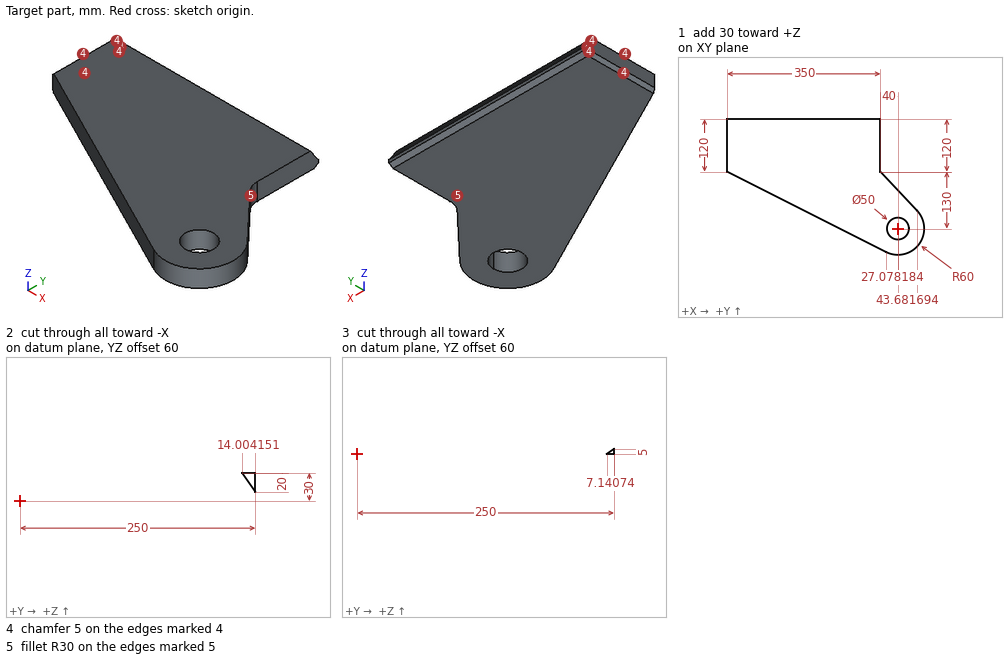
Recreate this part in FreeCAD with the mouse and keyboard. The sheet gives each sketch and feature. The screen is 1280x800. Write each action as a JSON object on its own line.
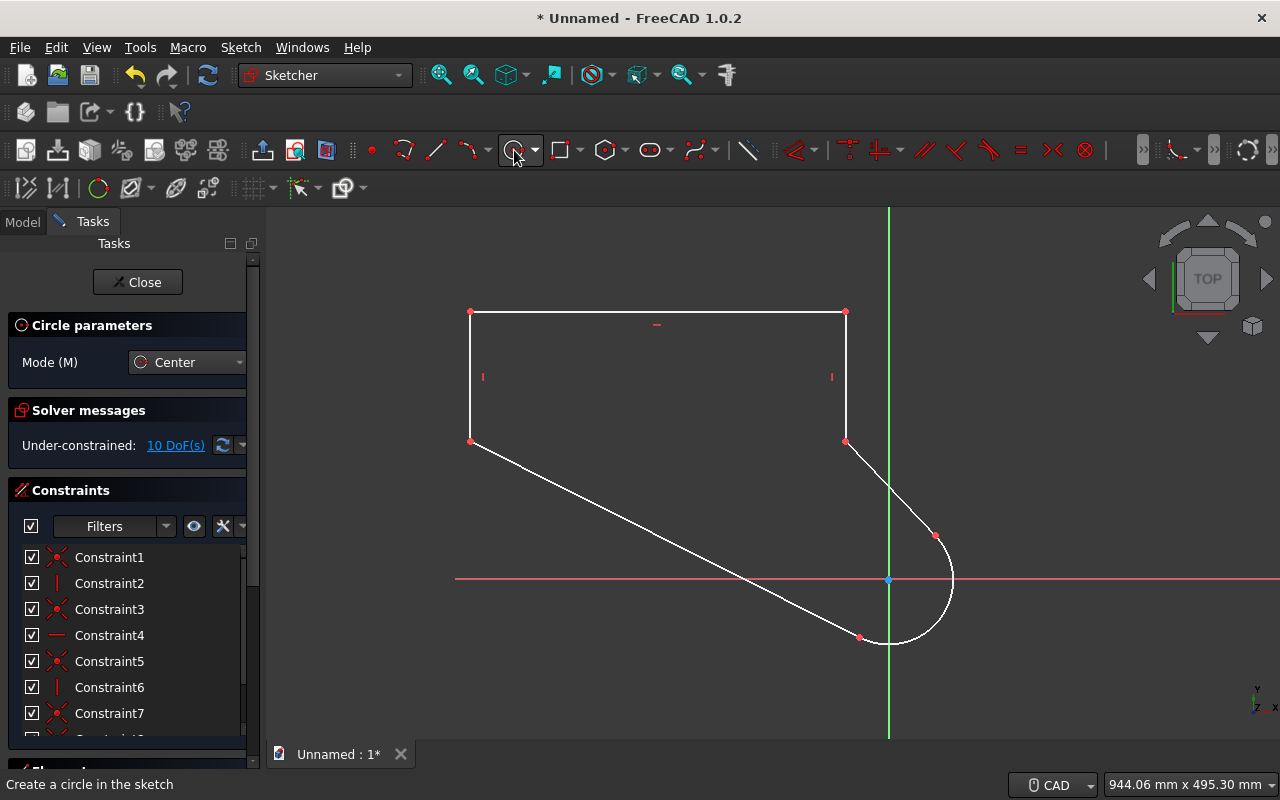
{"action": "left_click", "coordinate": [889, 579]}
{"action": "mouse_move", "coordinate": [908, 560]}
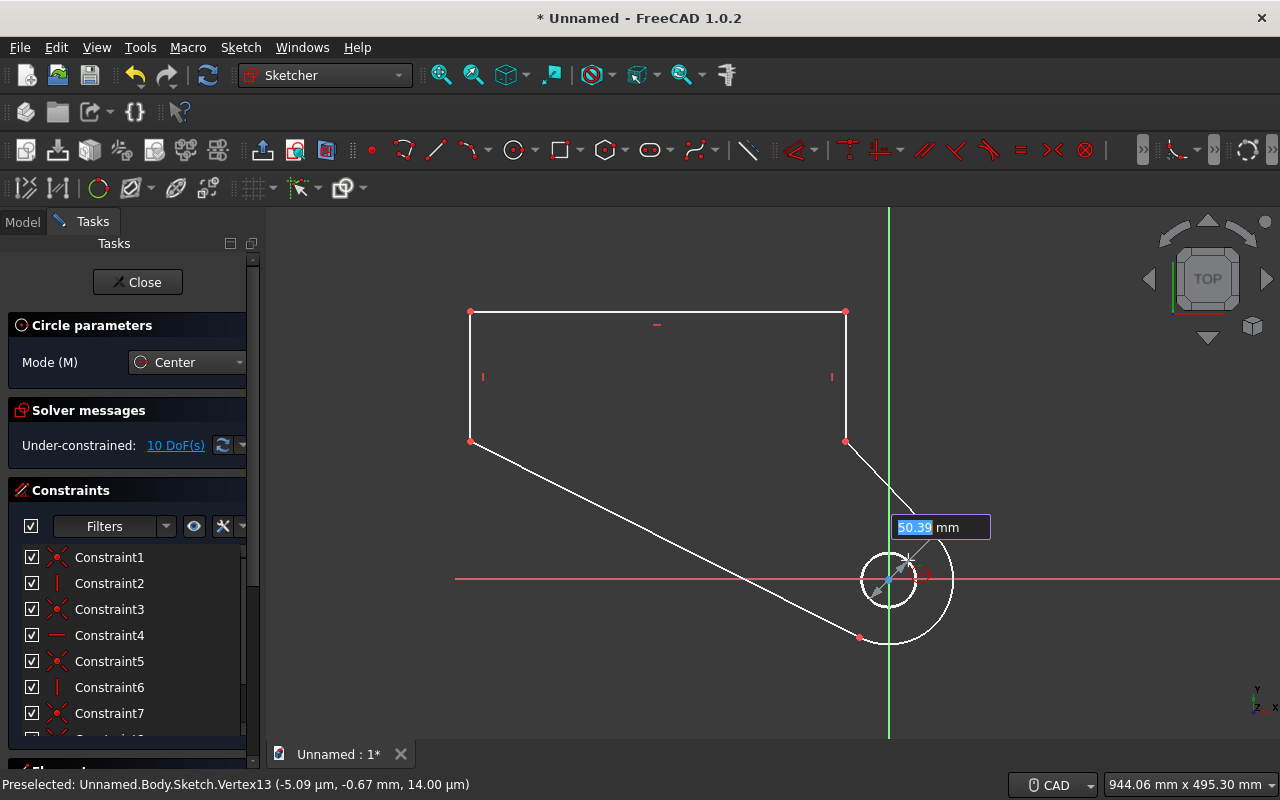
{"action": "type", "text": "50"}
{"action": "key", "text": "Return"}
{"action": "key", "text": "Escape"}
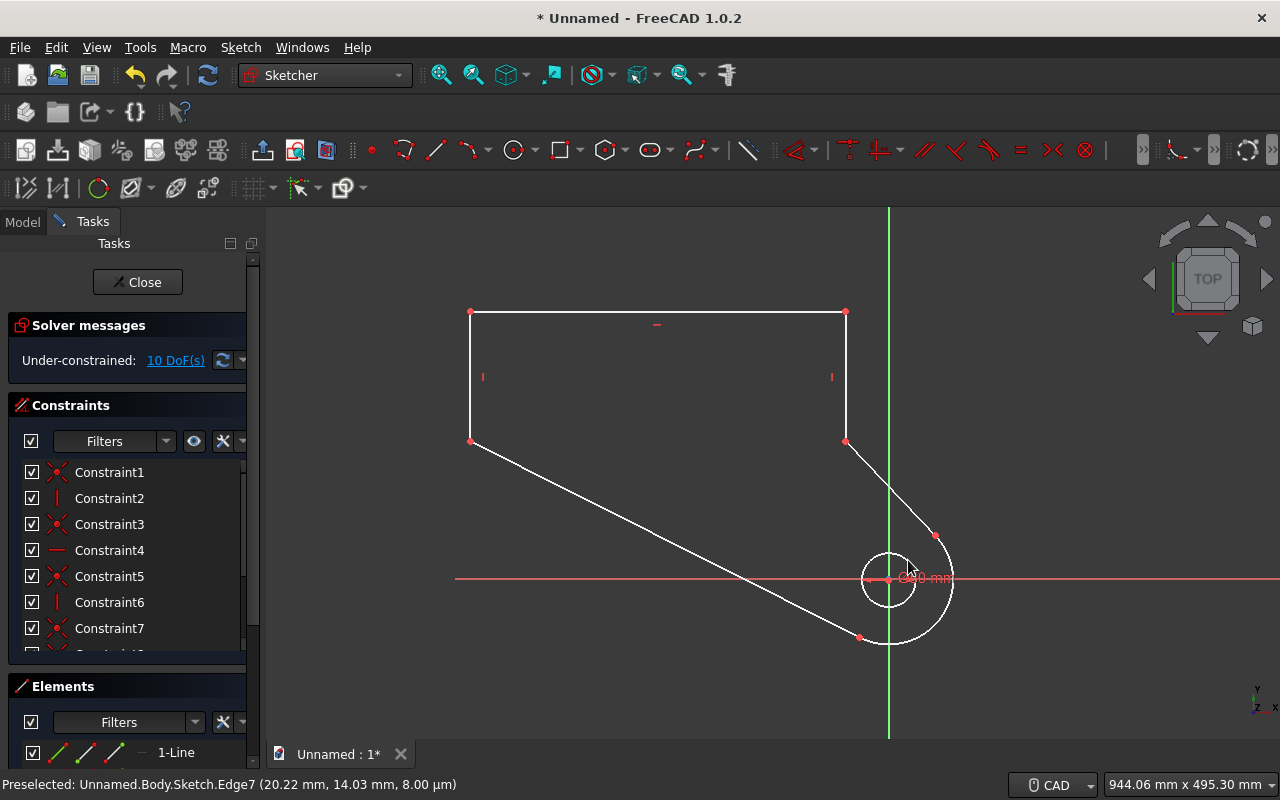
{"action": "scroll", "coordinate": [889, 580], "scroll_direction": "up", "scroll_amount": 2}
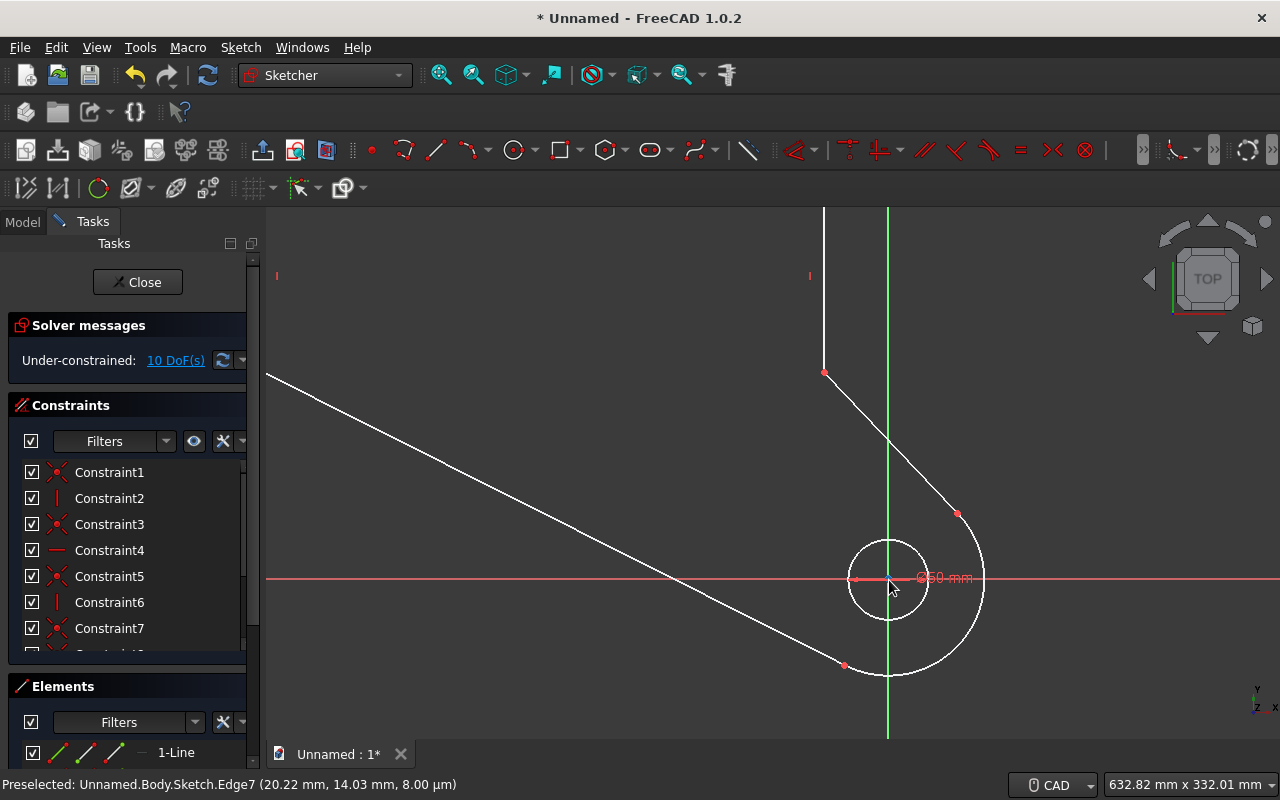
{"action": "left_click_drag", "start_coordinate": [878, 569], "coordinate": [898, 590]}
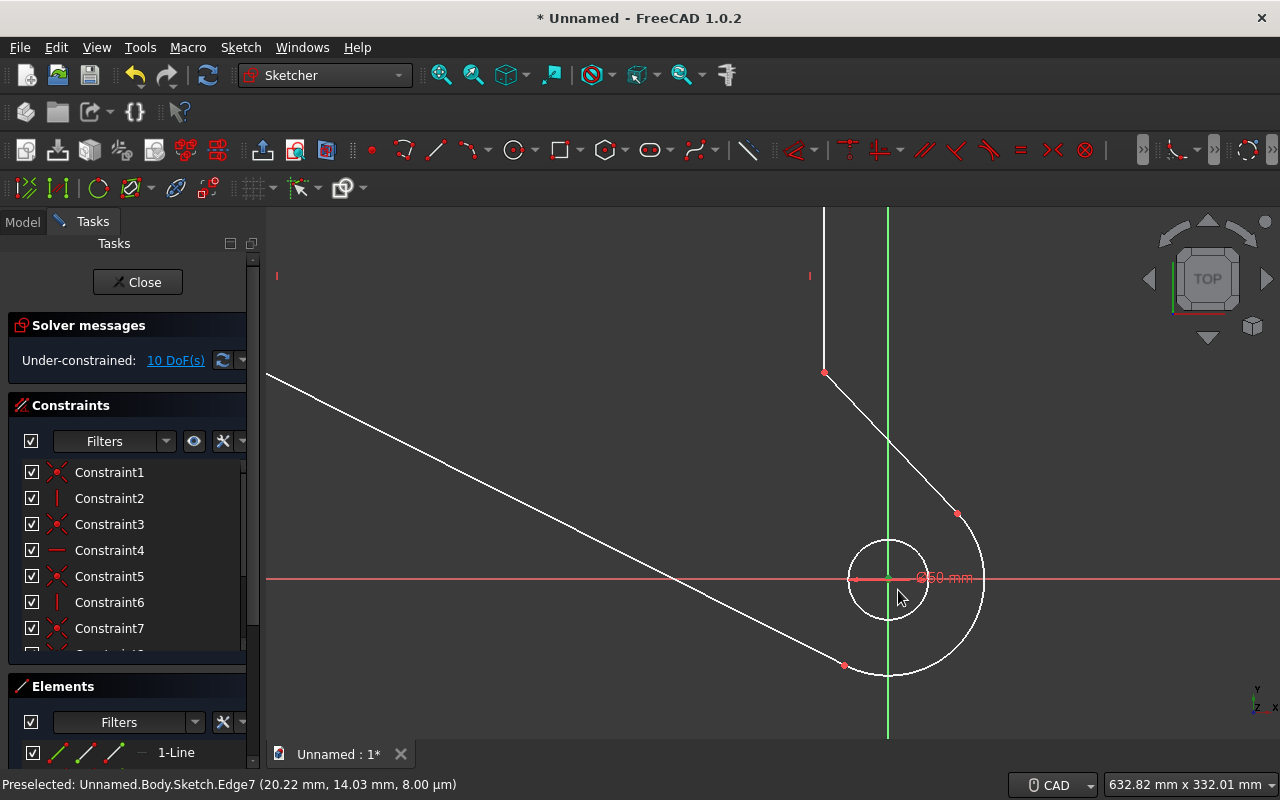
{"action": "key", "text": "c"}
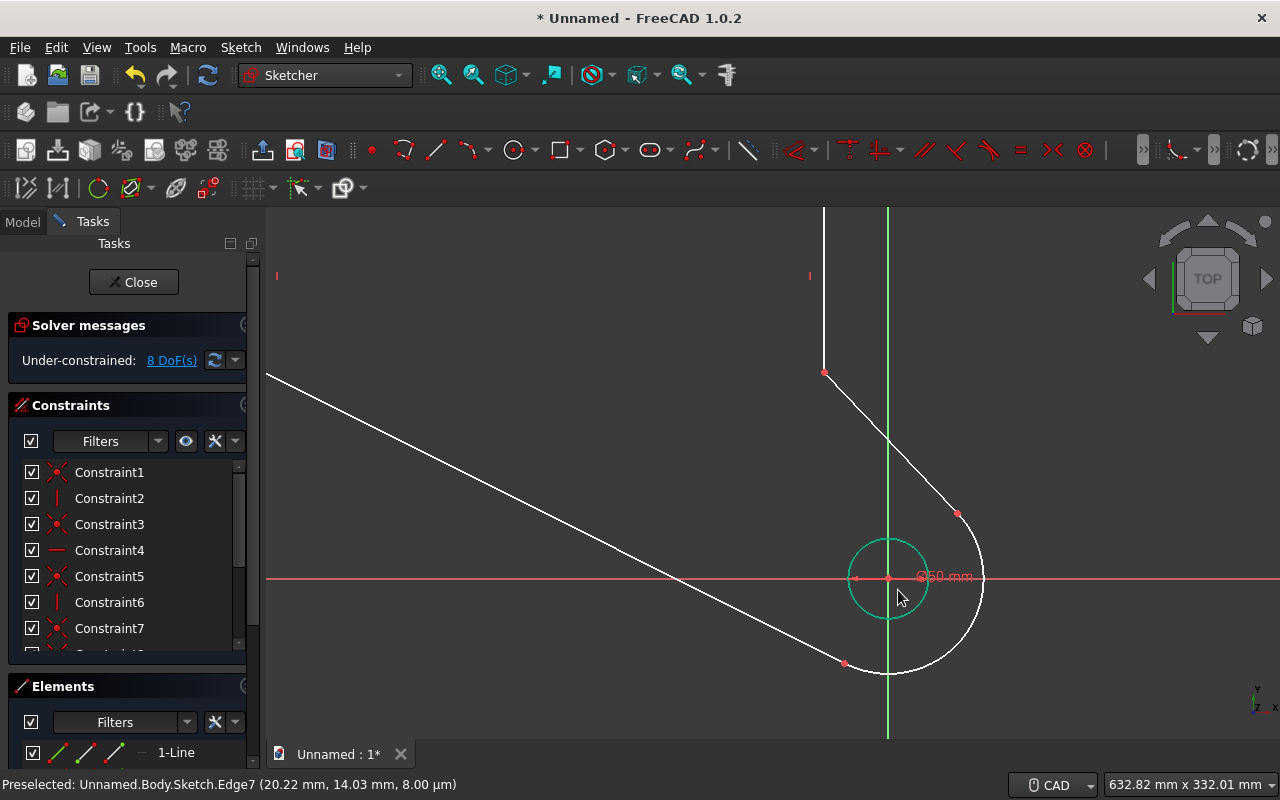
{"action": "key", "text": "d"}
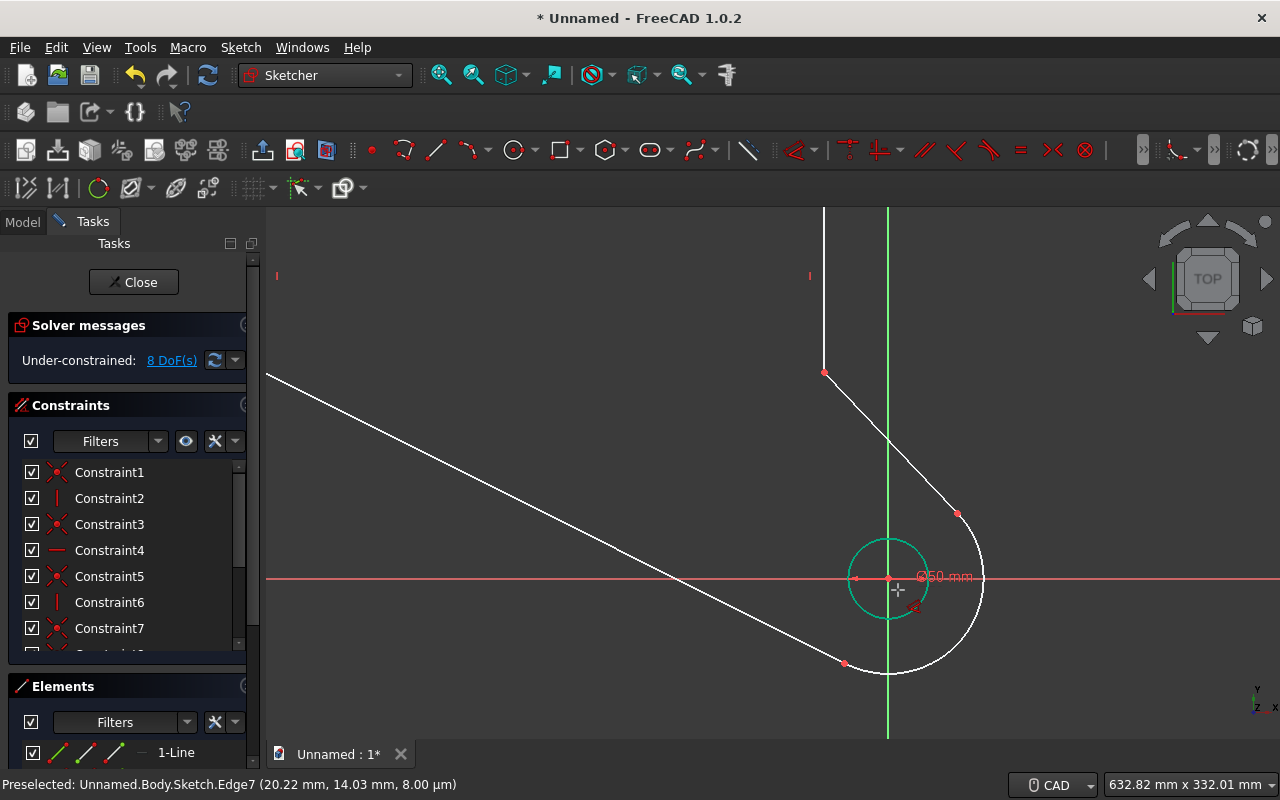
{"action": "left_click", "coordinate": [922, 668]}
{"action": "left_click", "coordinate": [933, 698]}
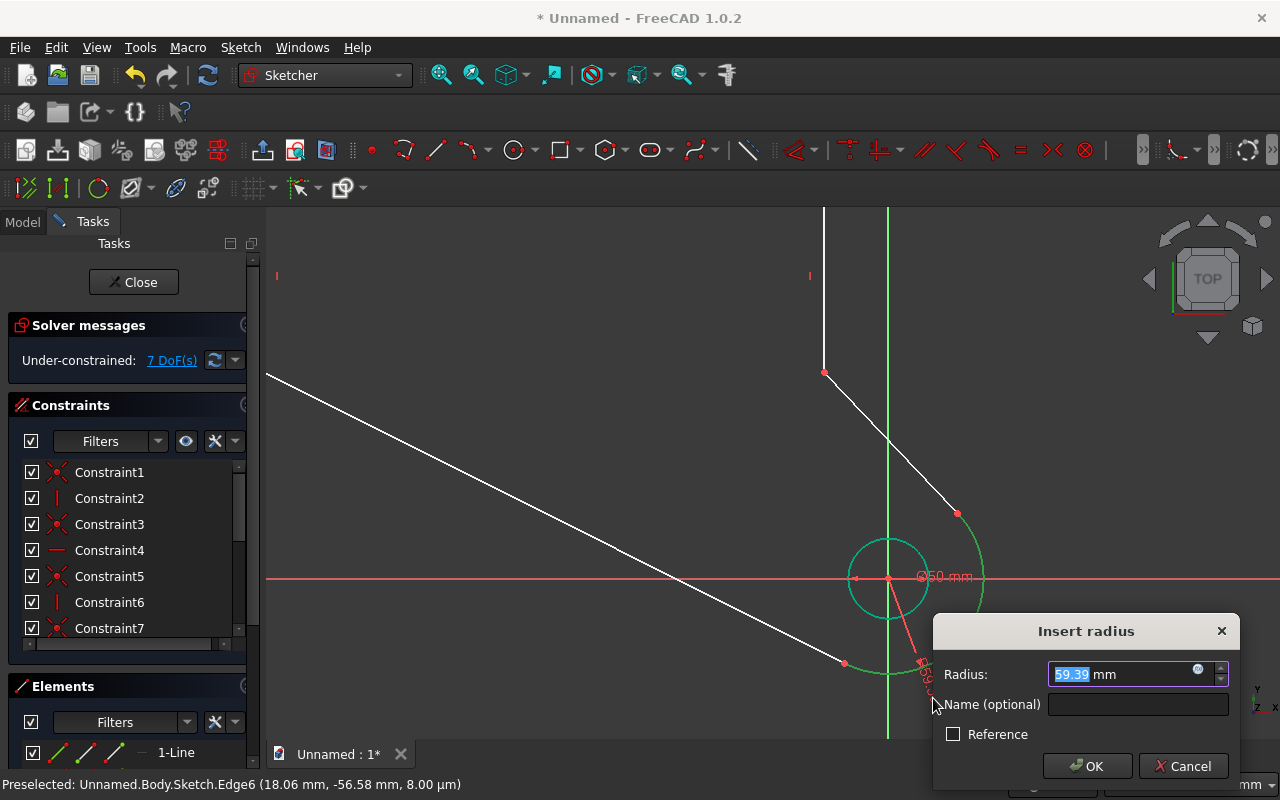
{"action": "type", "text": "60"}
{"action": "key", "text": "Return"}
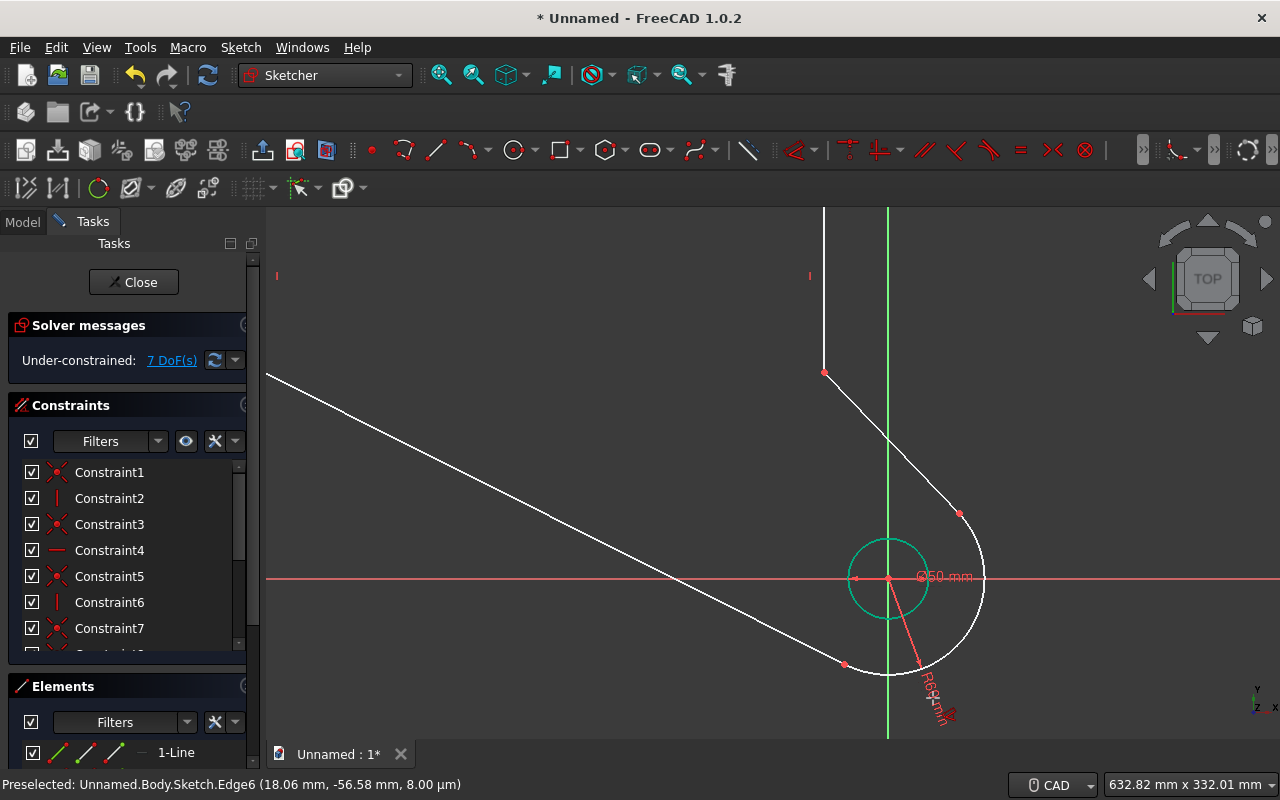
{"action": "left_click", "coordinate": [824, 315]}
{"action": "left_click", "coordinate": [858, 304]}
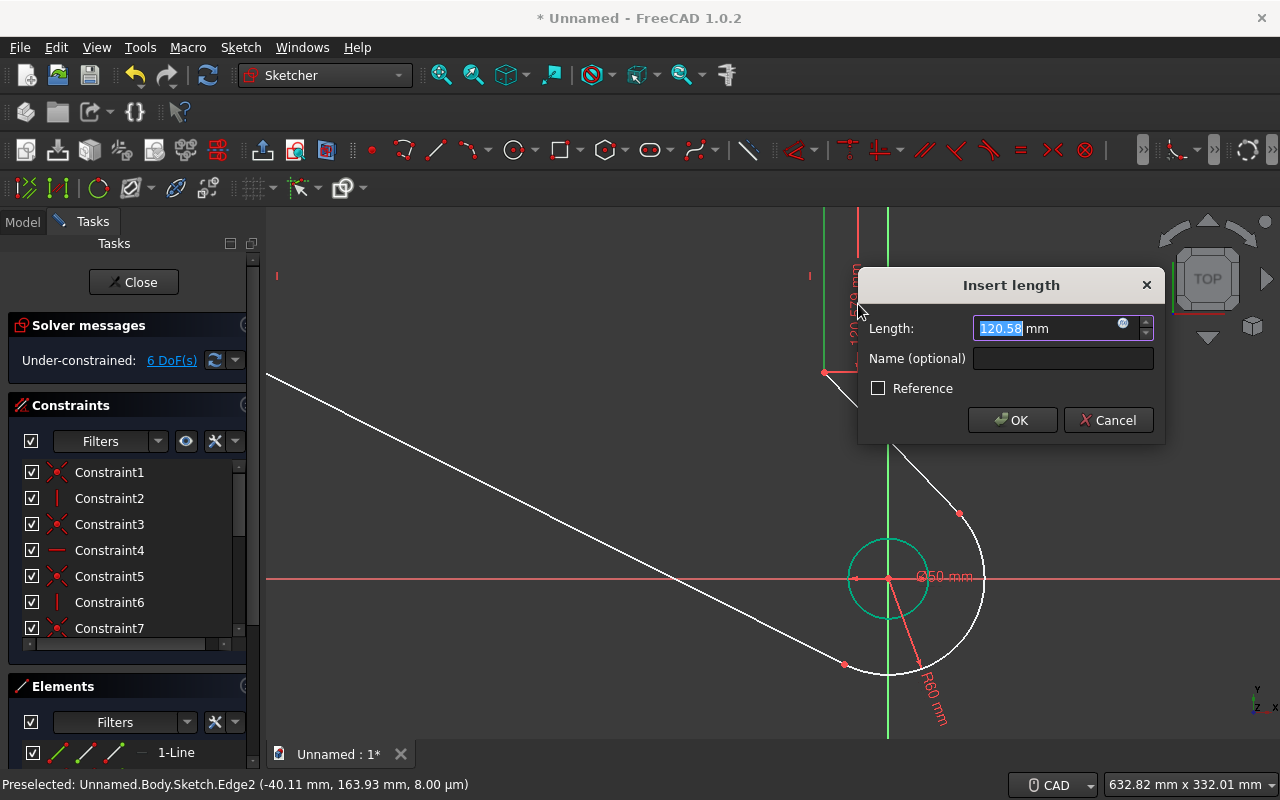
{"action": "type", "text": "120"}
{"action": "key", "text": "Return"}